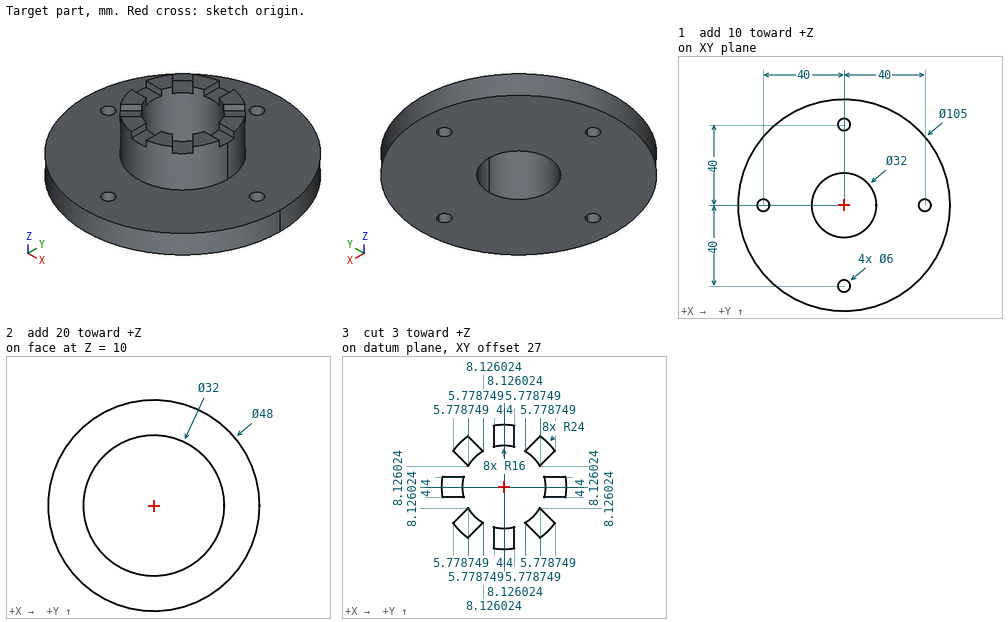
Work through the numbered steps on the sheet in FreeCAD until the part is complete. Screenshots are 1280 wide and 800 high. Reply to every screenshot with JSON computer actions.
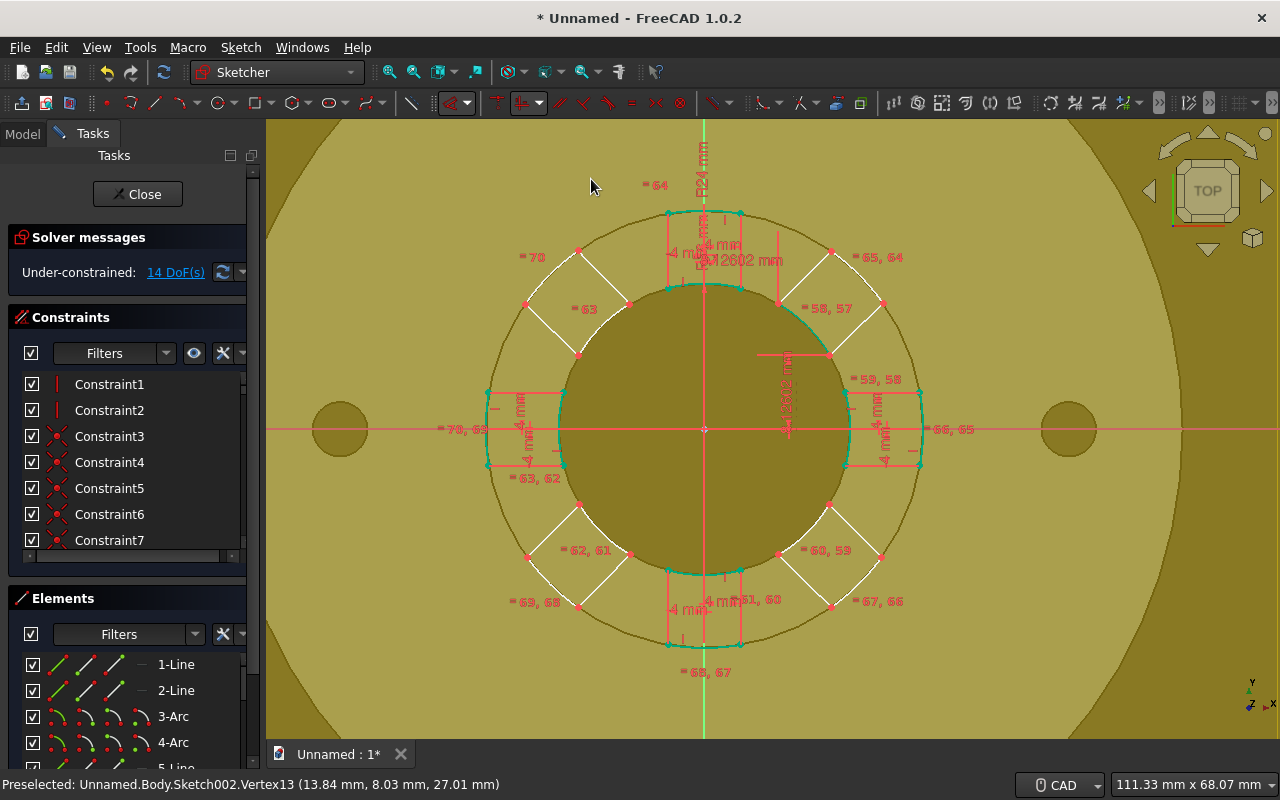
{"action": "left_click", "coordinate": [829, 504]}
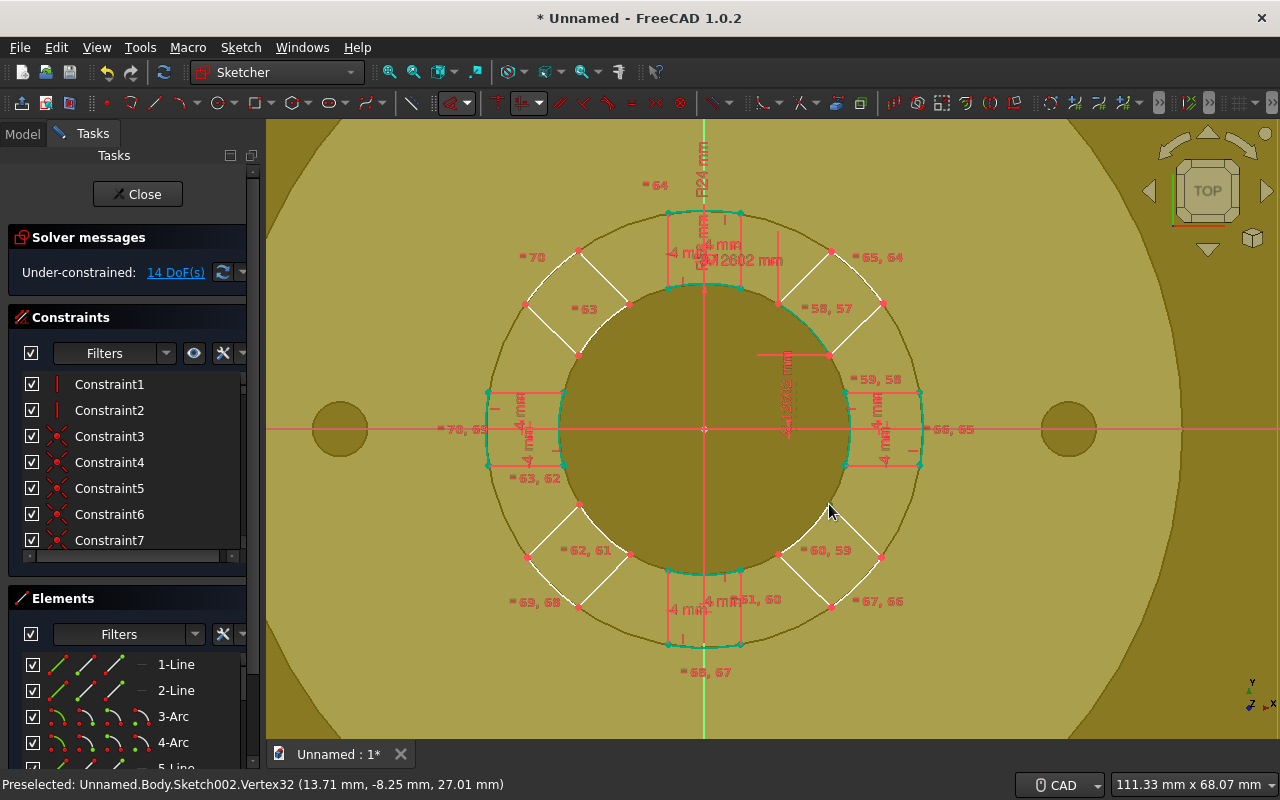
{"action": "left_click", "coordinate": [470, 104]}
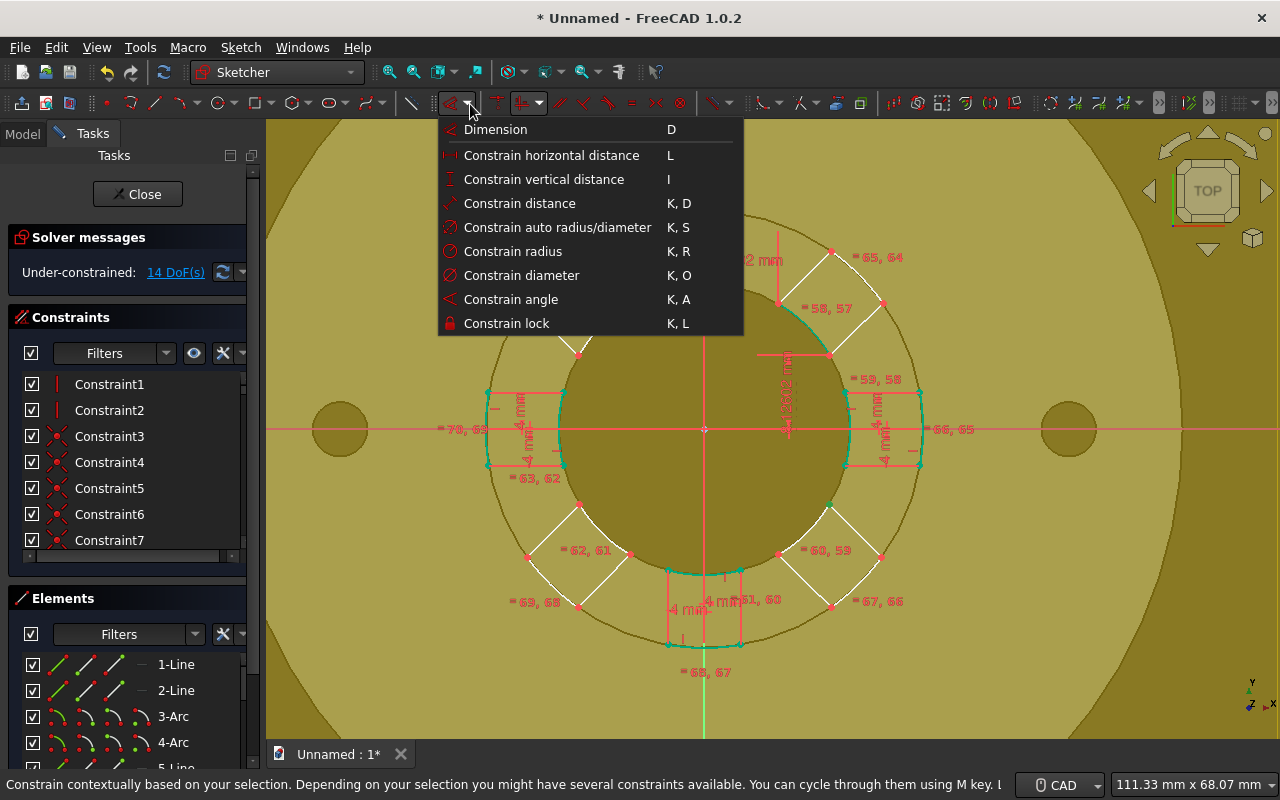
{"action": "left_click", "coordinate": [591, 179]}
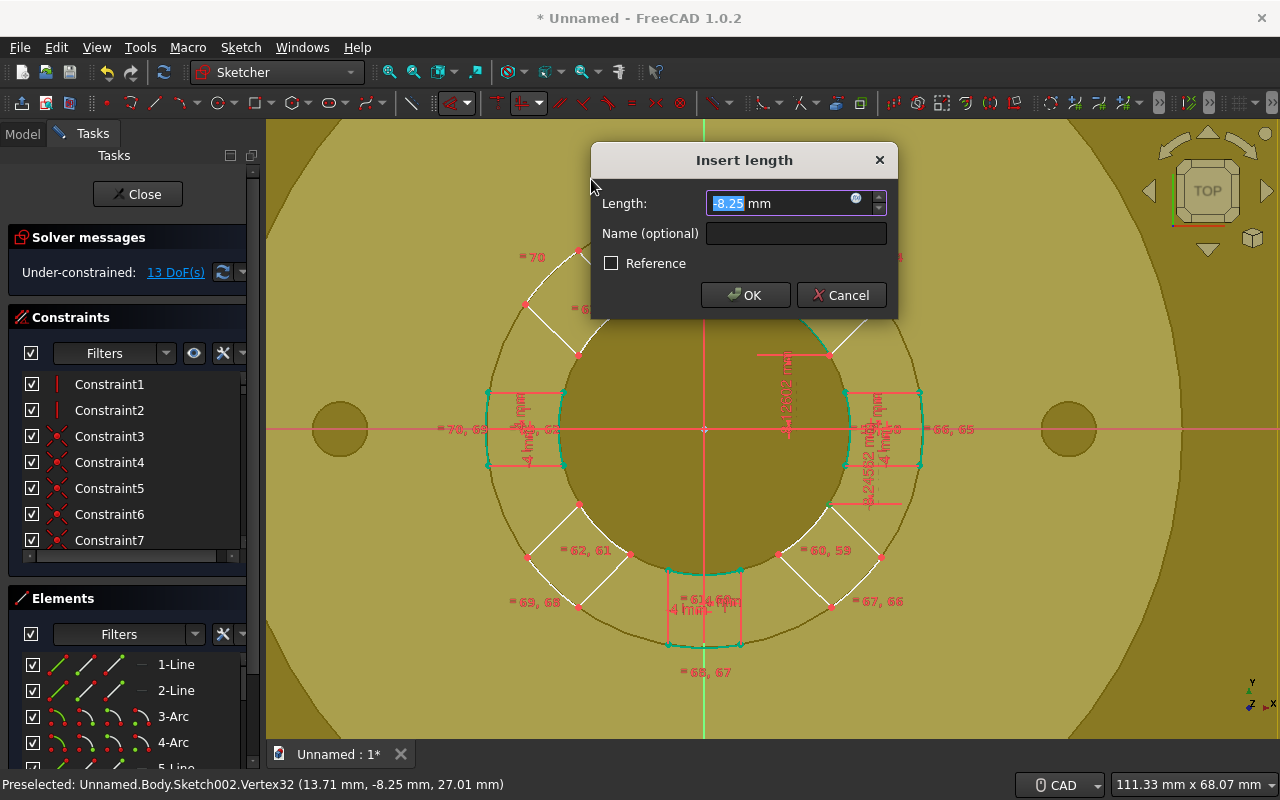
{"action": "type", "text": "-8.126024"}
{"action": "key", "text": "Return"}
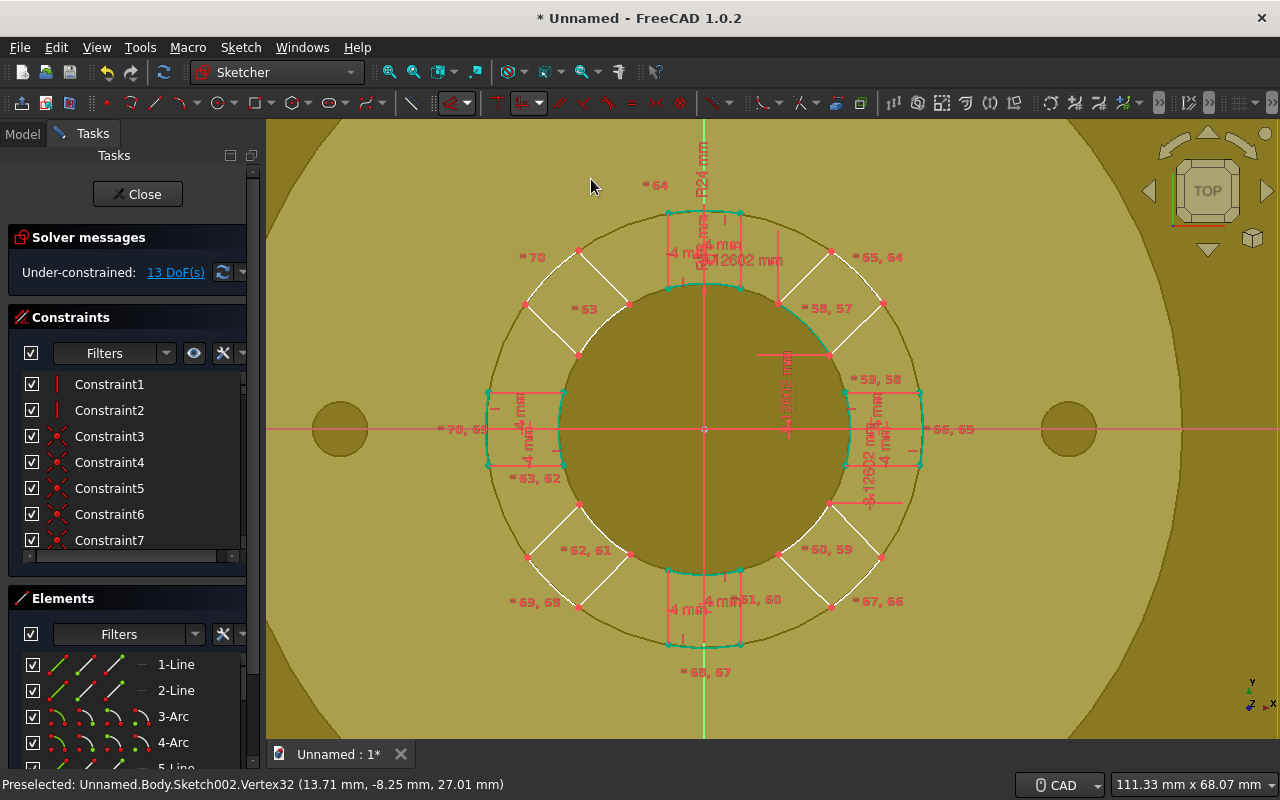
{"action": "left_click", "coordinate": [778, 555]}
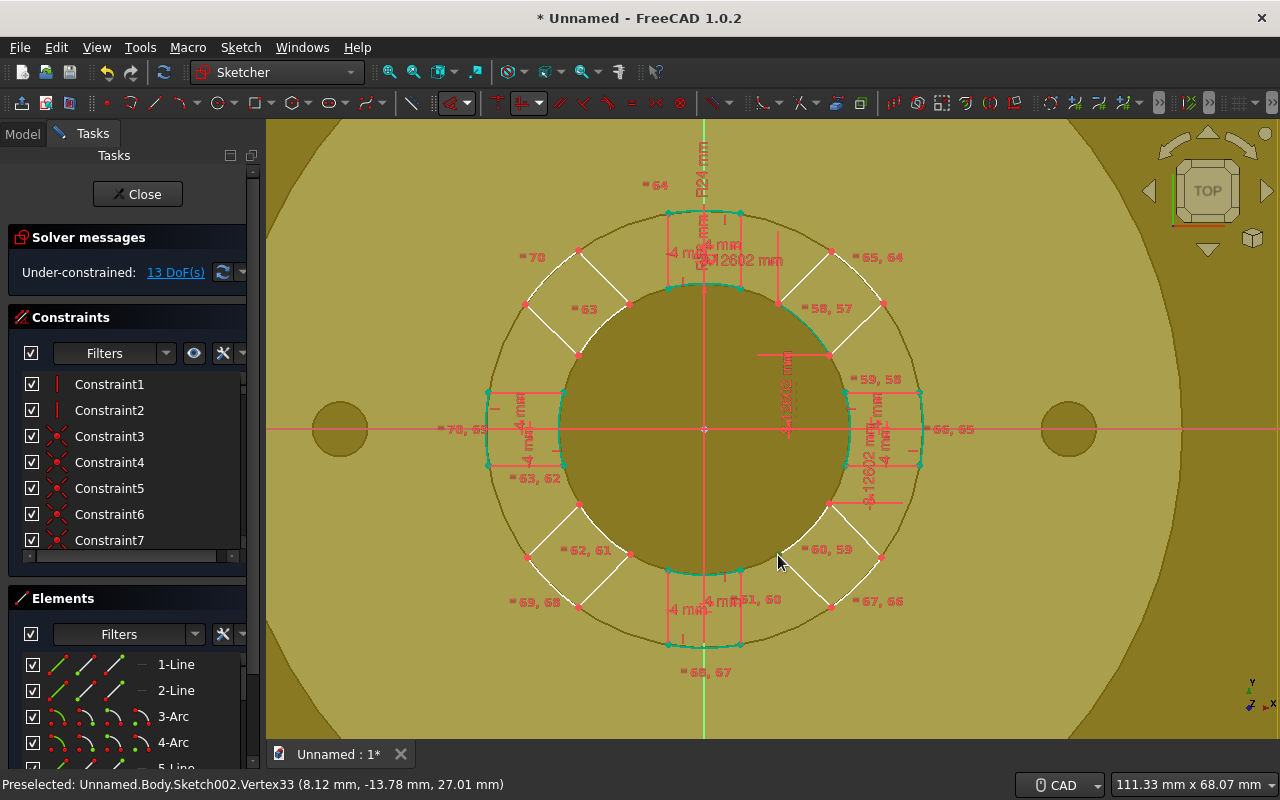
{"action": "key", "text": "l"}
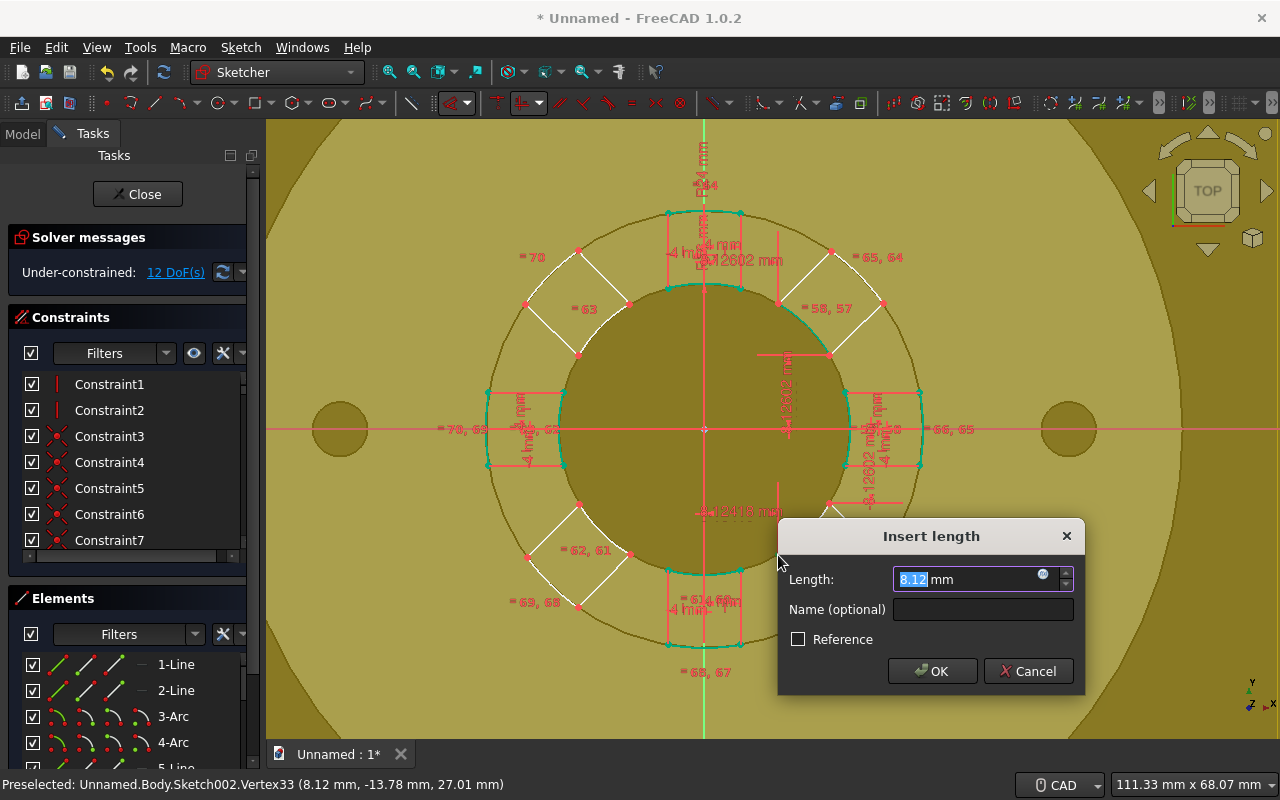
{"action": "type", "text": "8.126024"}
{"action": "key", "text": "Return"}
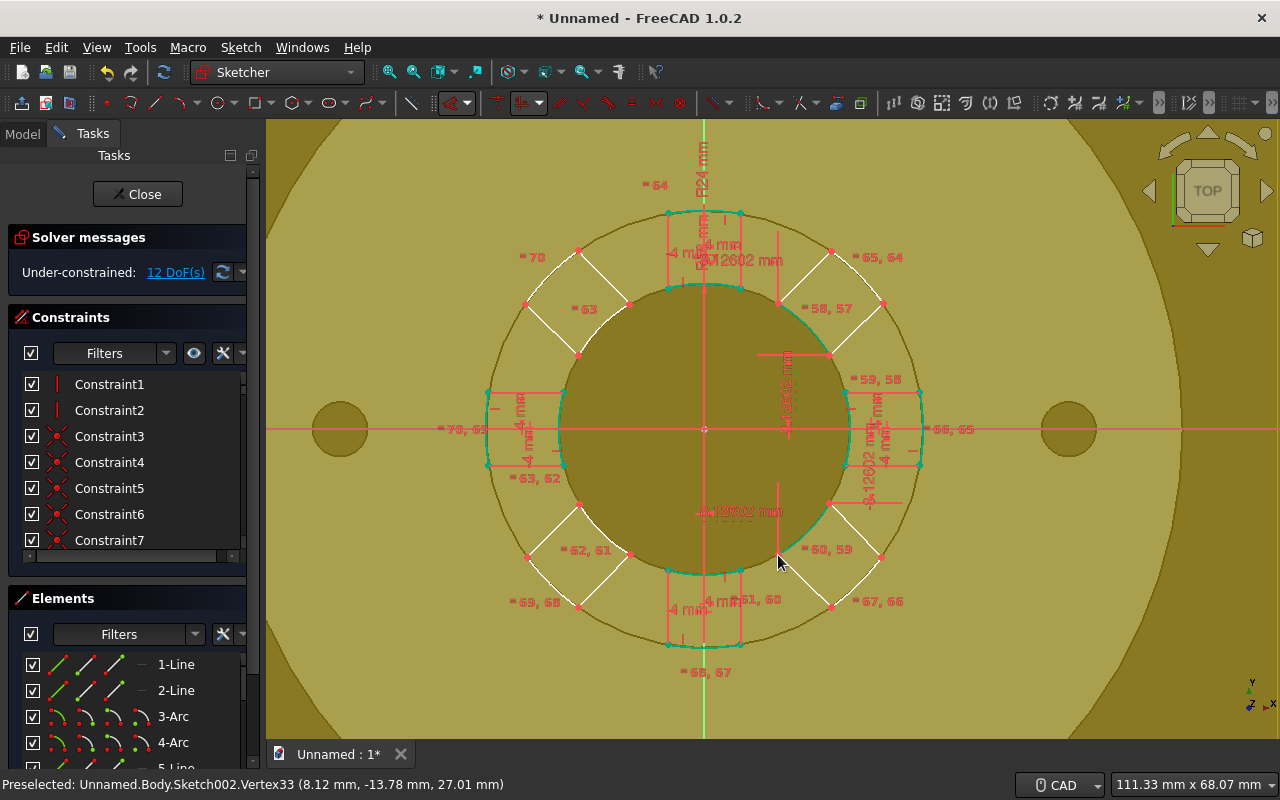
{"action": "left_click", "coordinate": [630, 555]}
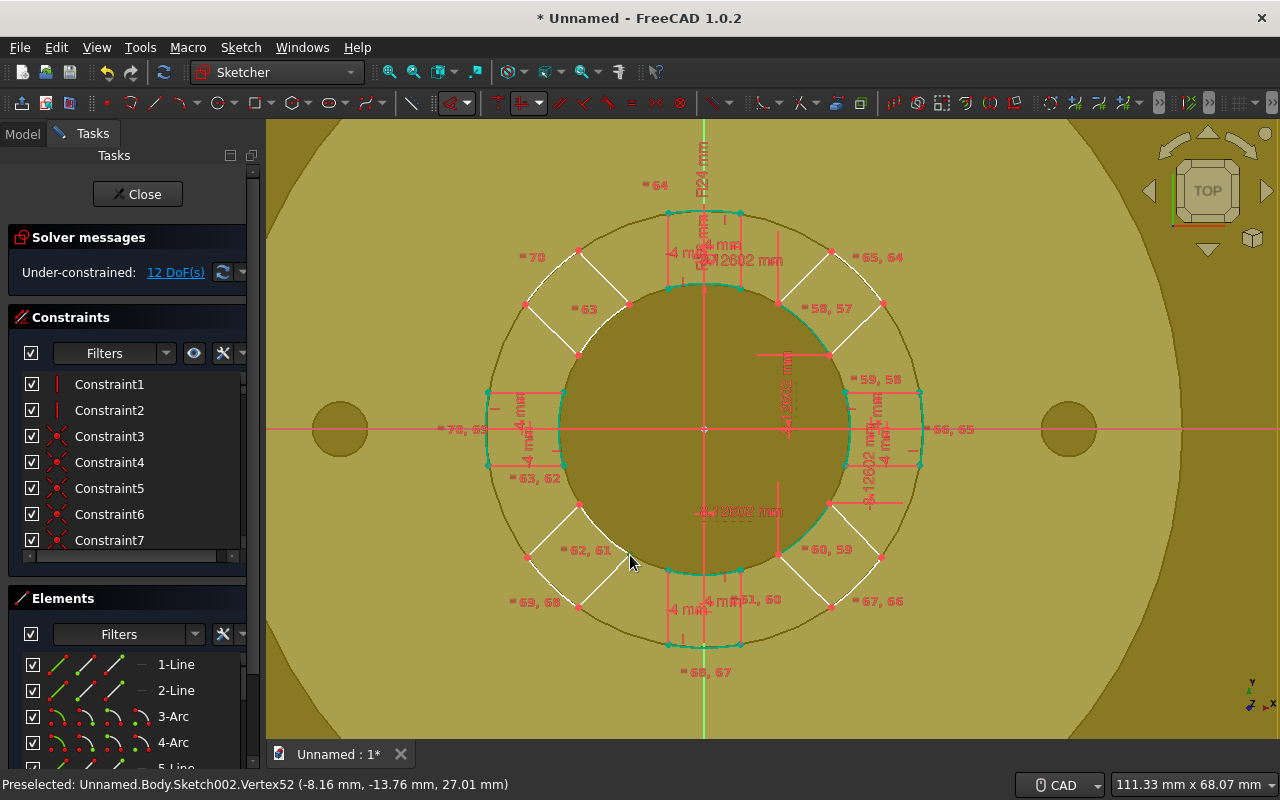
{"action": "left_click", "coordinate": [470, 104]}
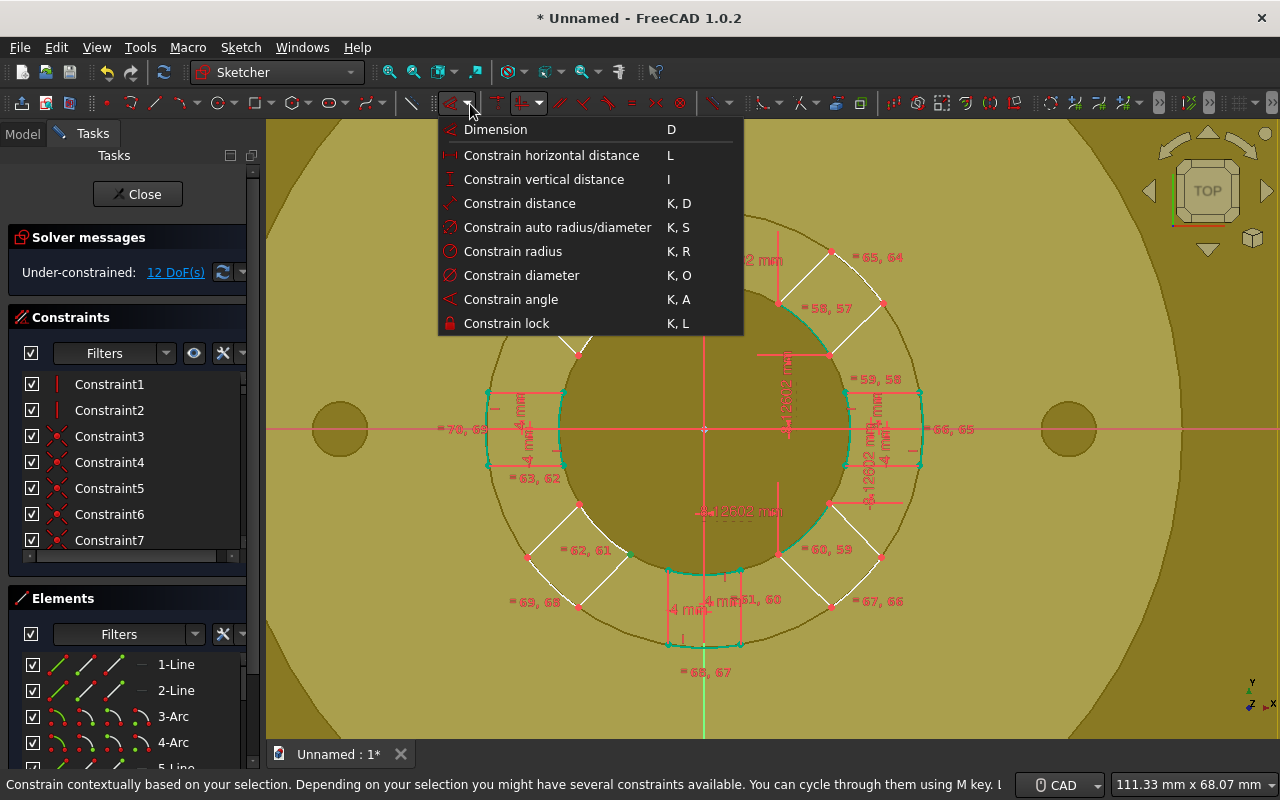
{"action": "left_click", "coordinate": [591, 155]}